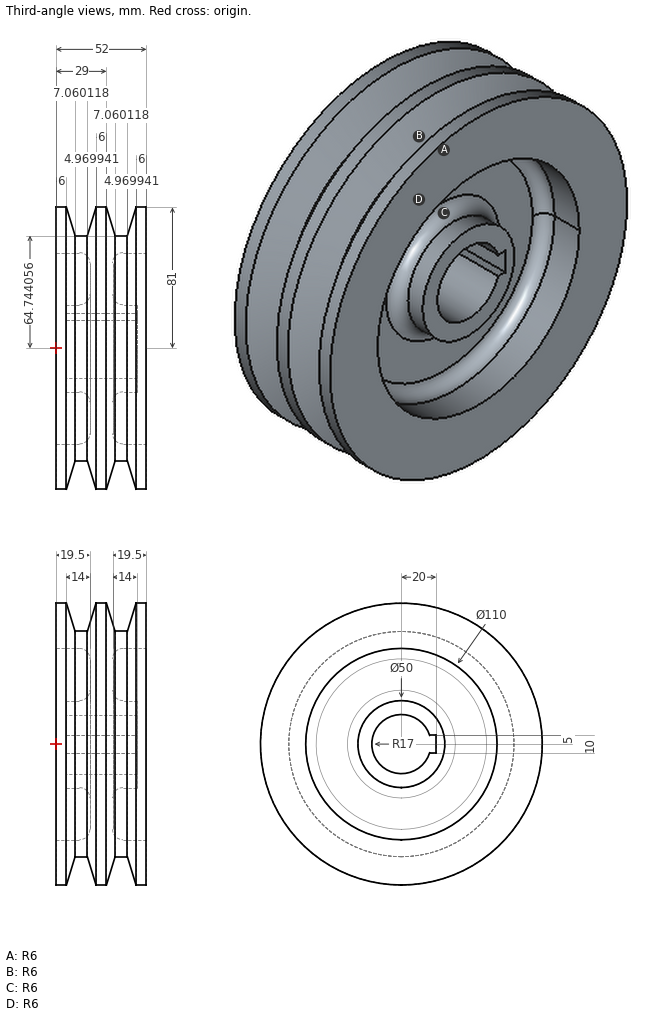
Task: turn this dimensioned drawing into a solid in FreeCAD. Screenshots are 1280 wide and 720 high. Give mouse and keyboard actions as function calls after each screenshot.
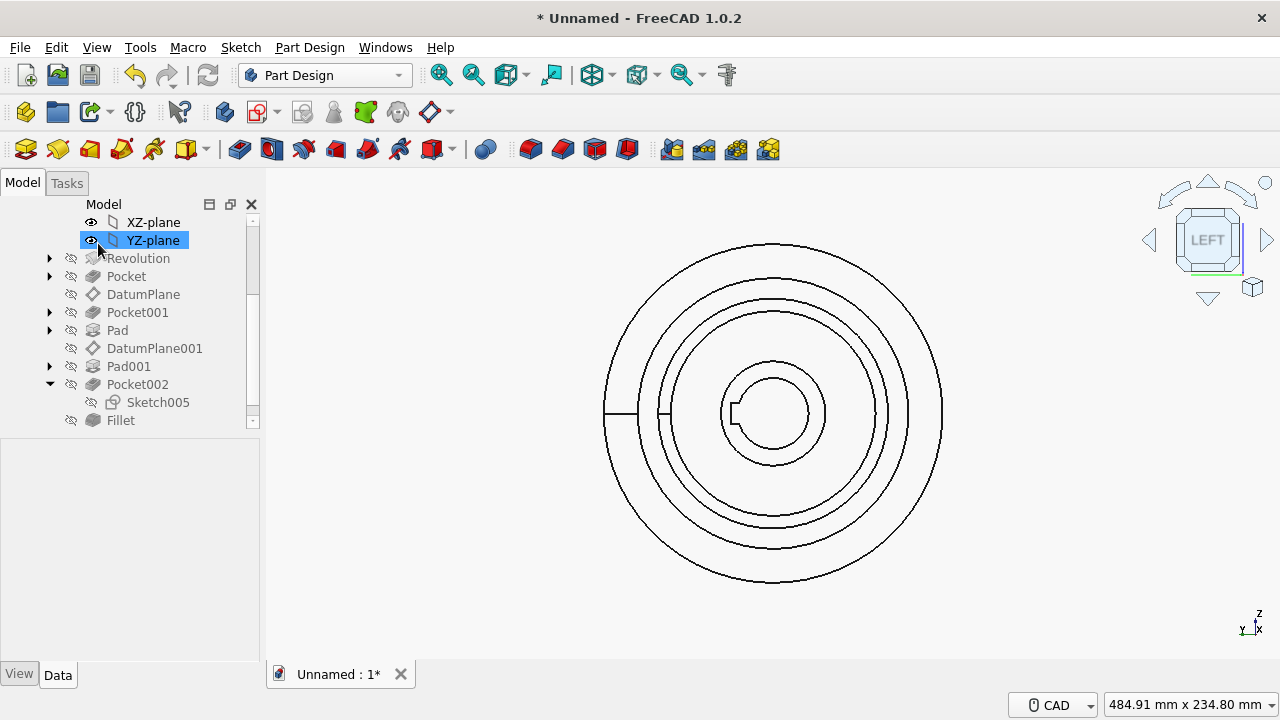
key(0)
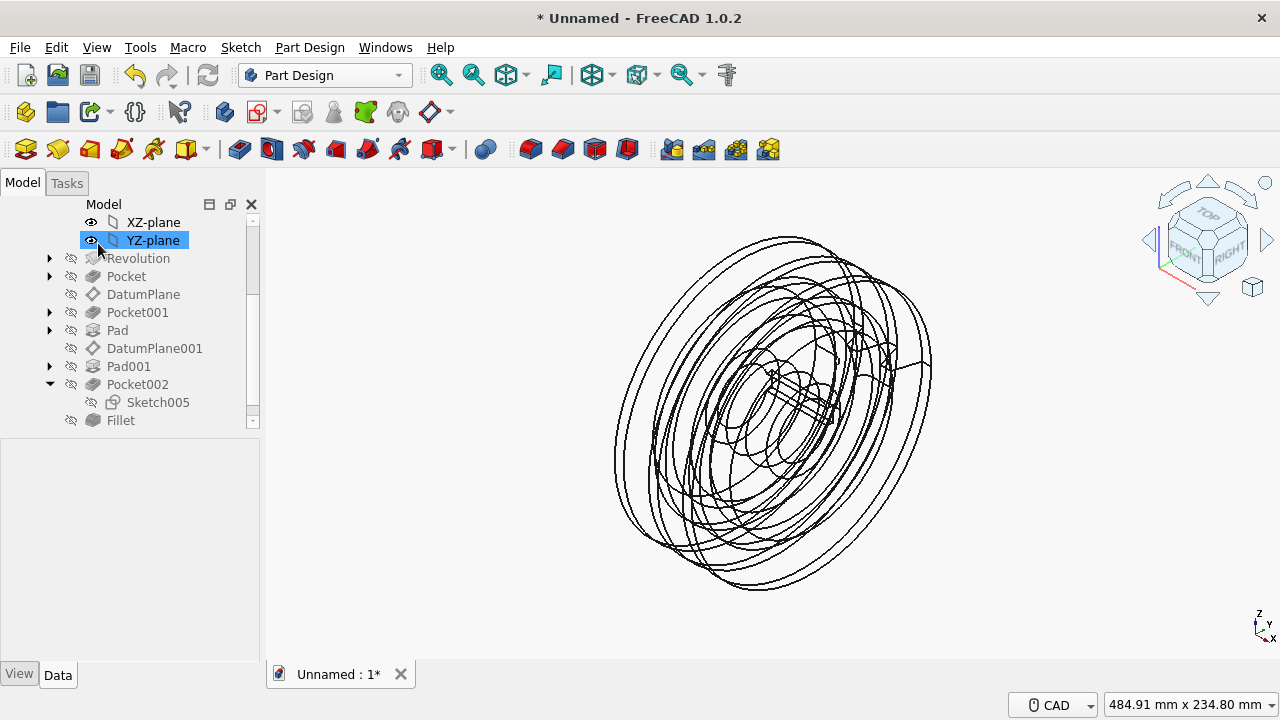
click(746, 439)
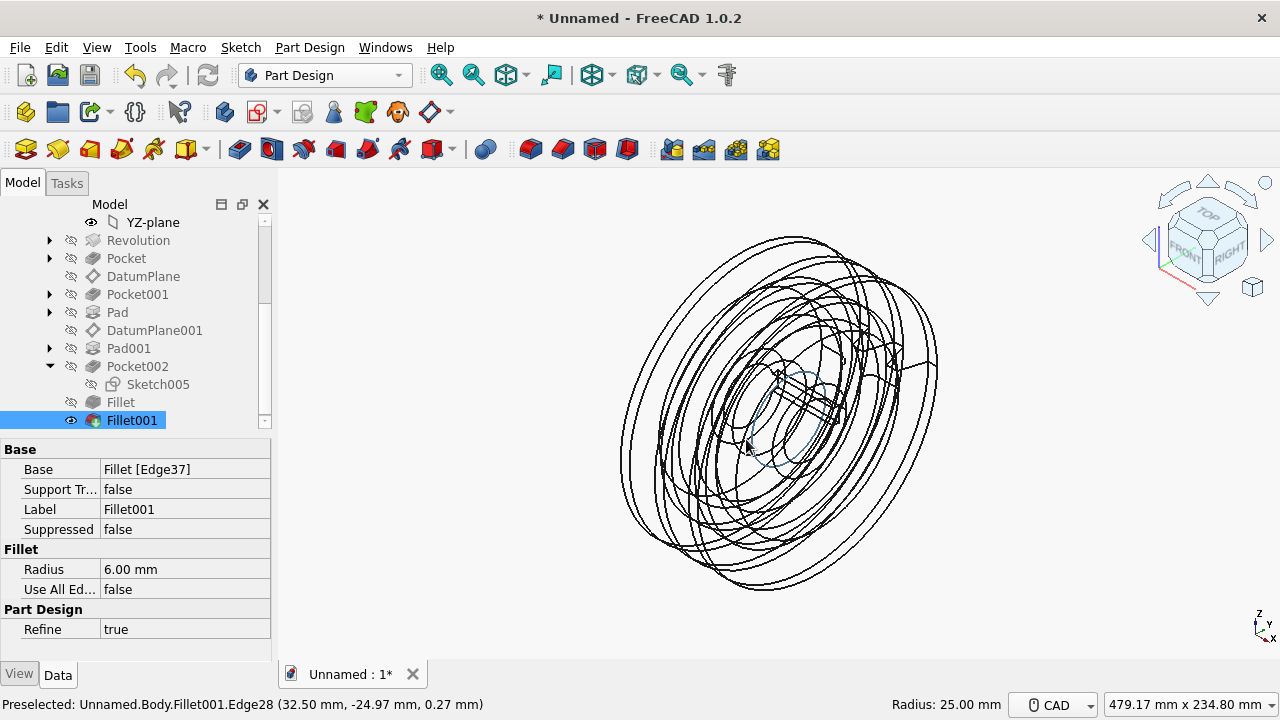
key(v)
key(1)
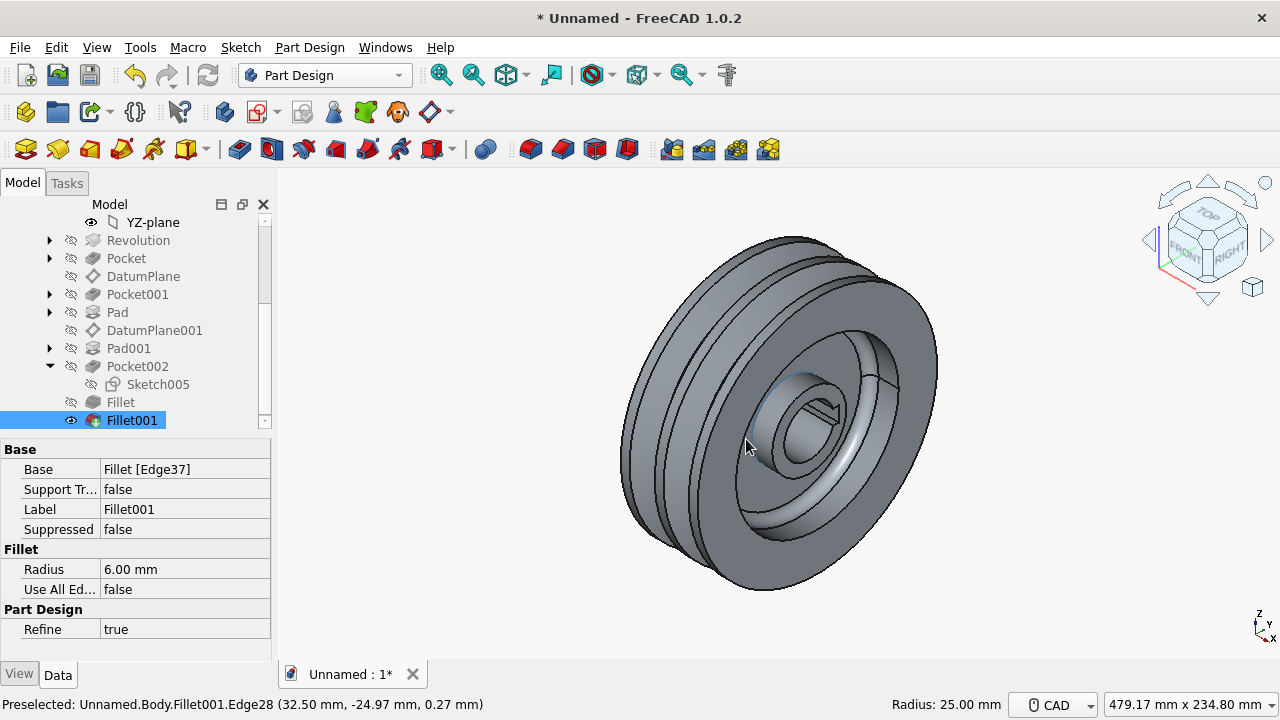
click(532, 150)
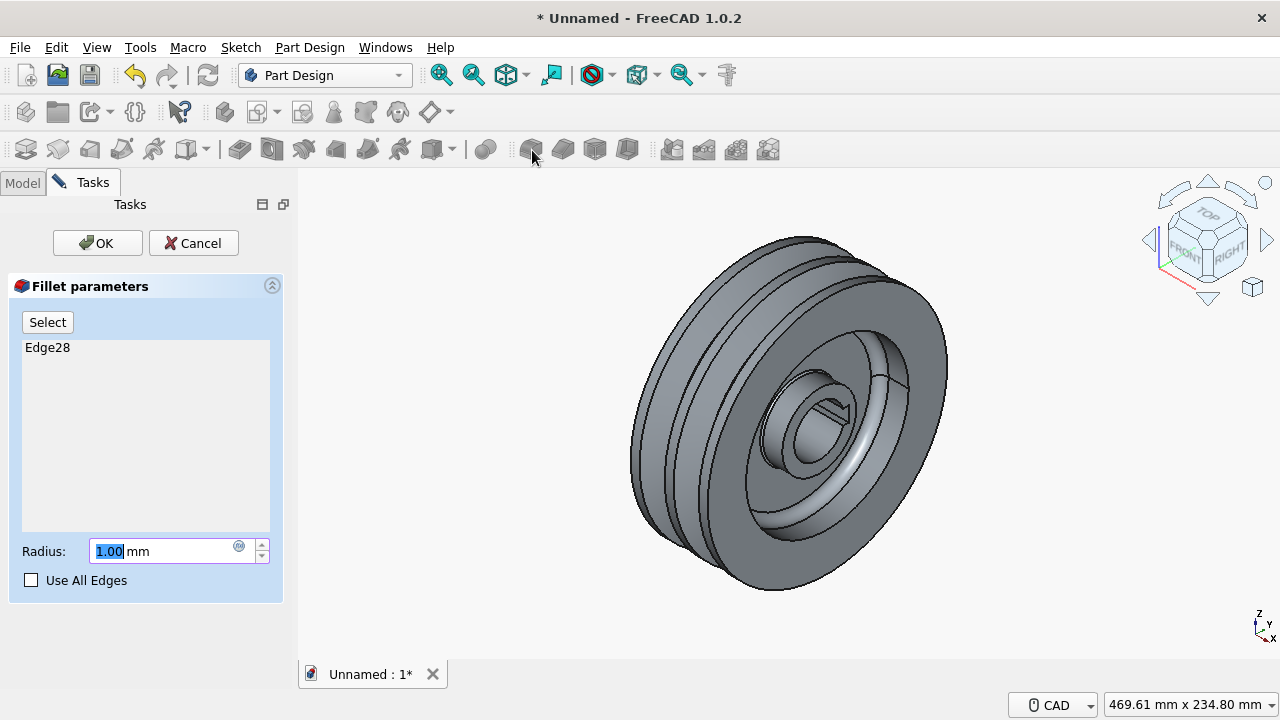
text(6)
key(Tab)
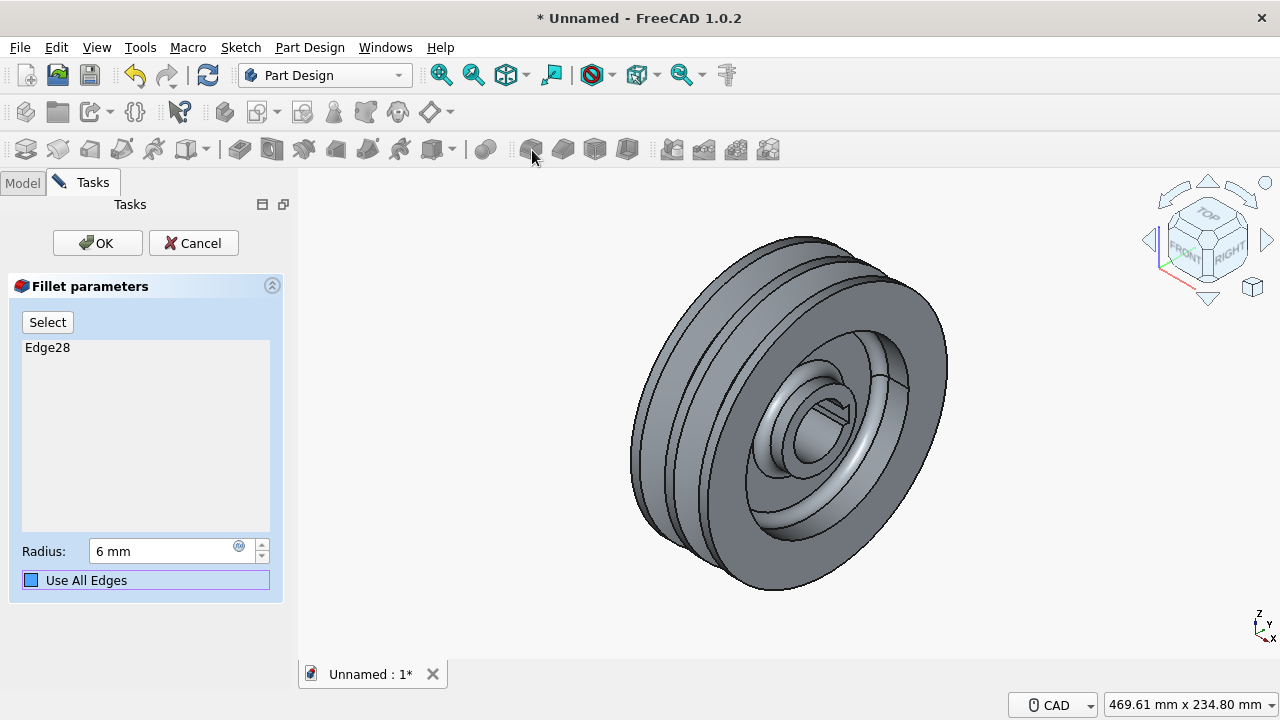
click(98, 243)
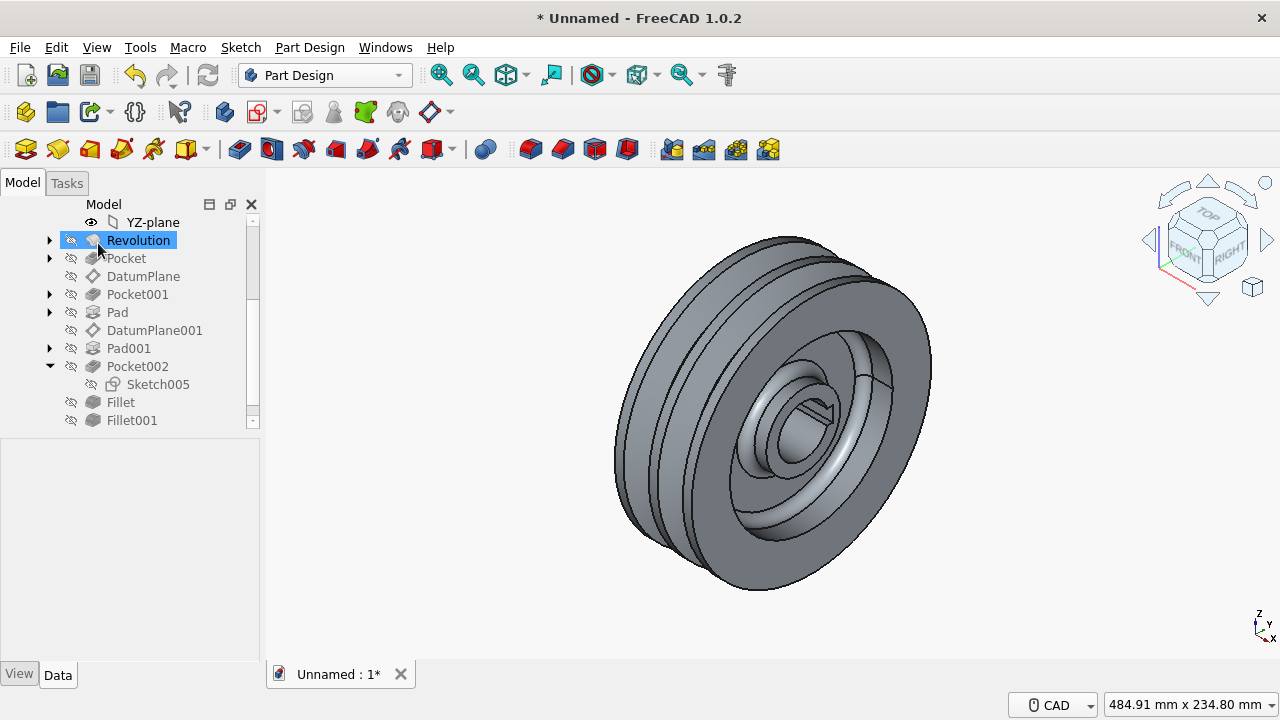
key(2)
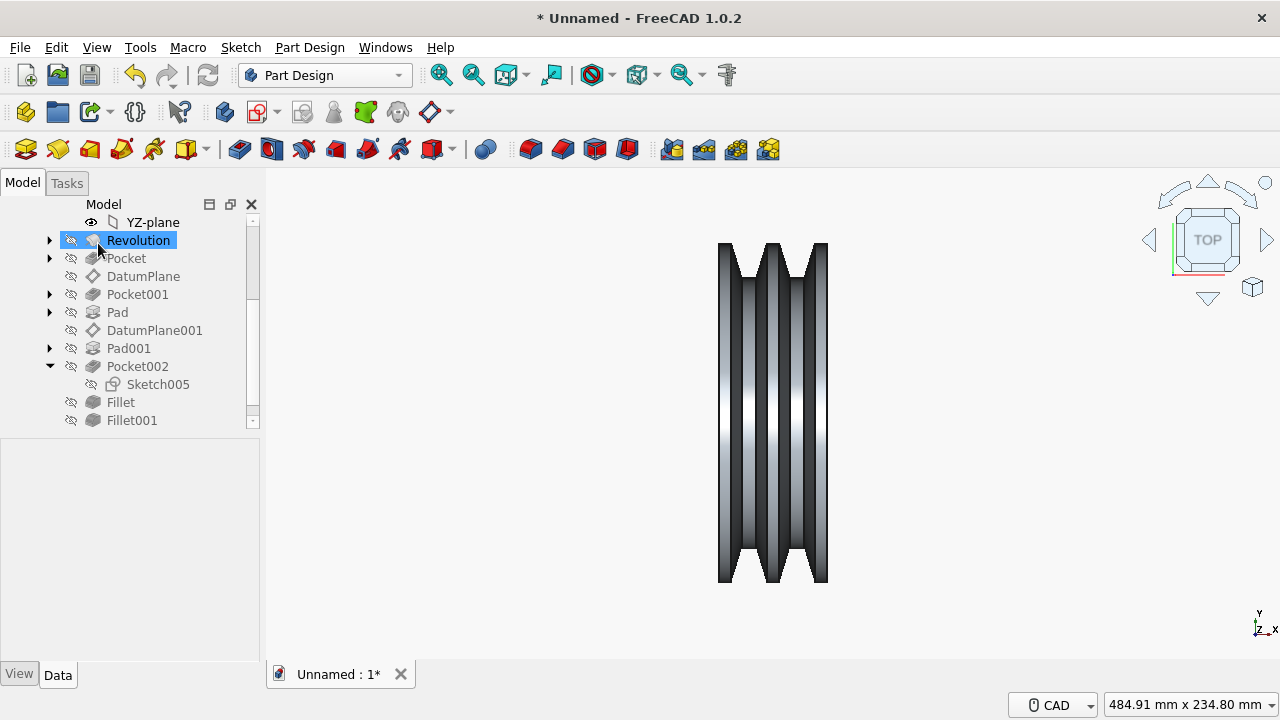
key(0)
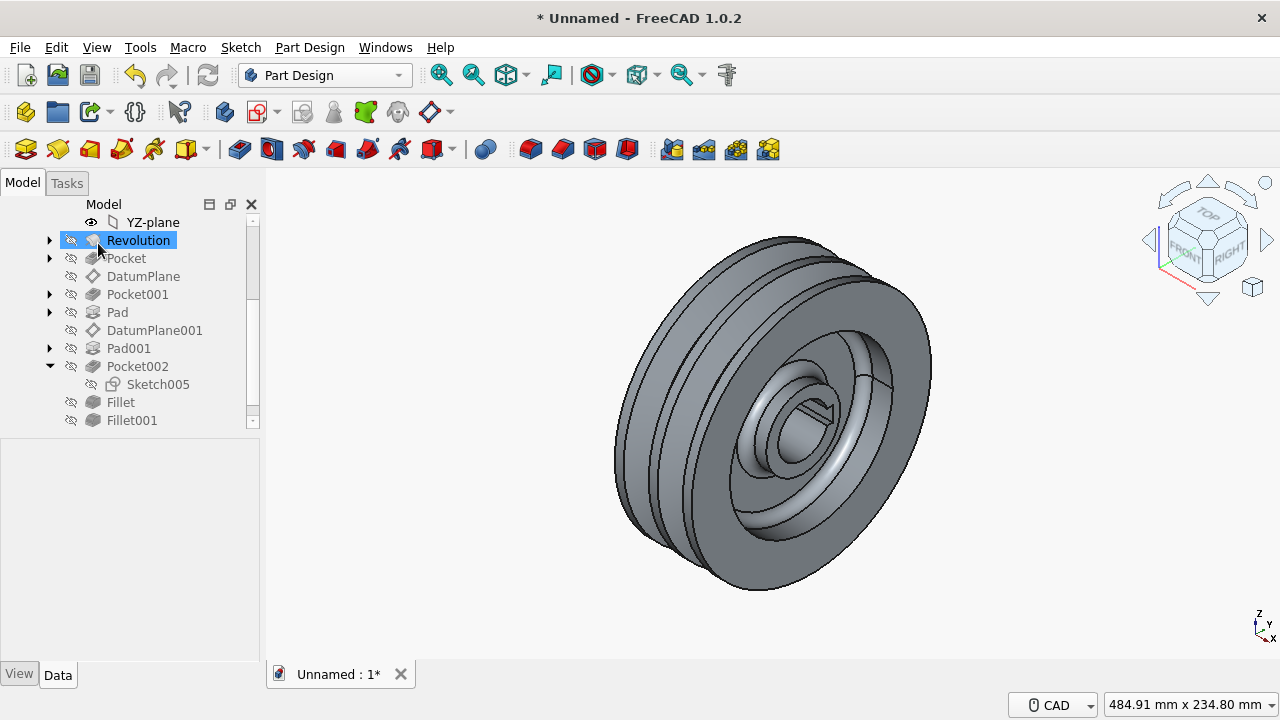
key(1)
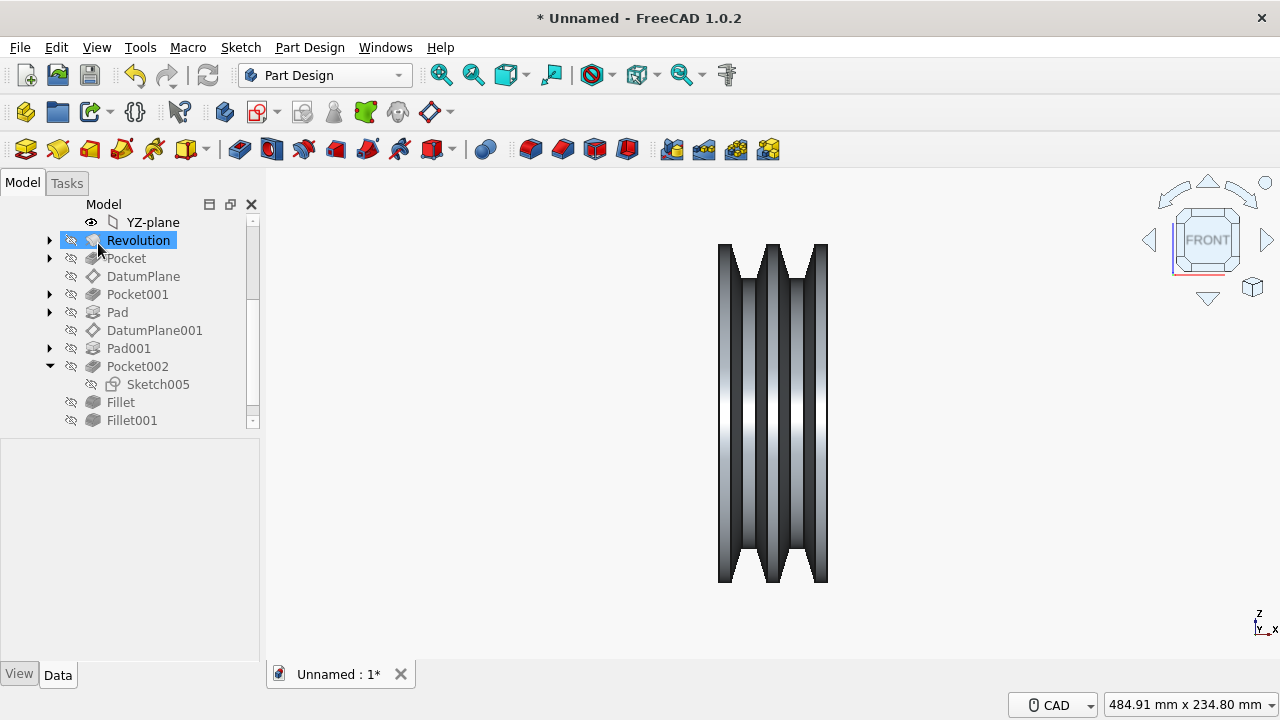
key(3)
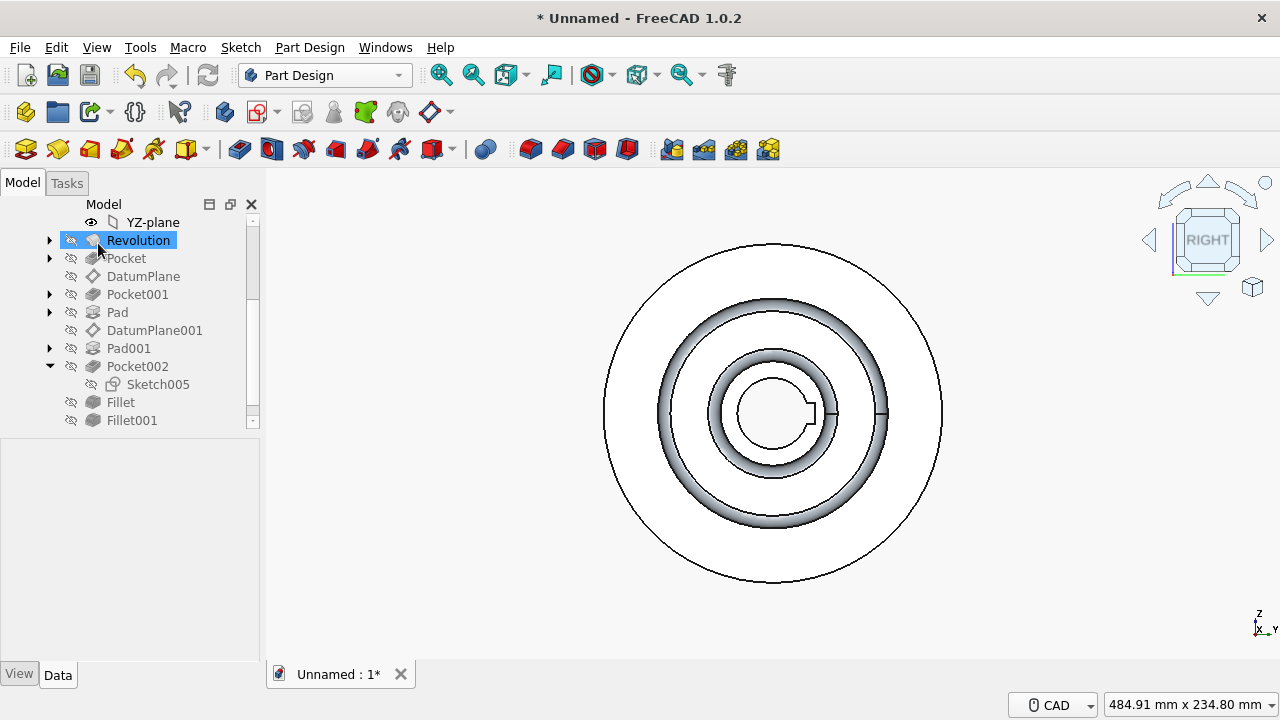
key(5)